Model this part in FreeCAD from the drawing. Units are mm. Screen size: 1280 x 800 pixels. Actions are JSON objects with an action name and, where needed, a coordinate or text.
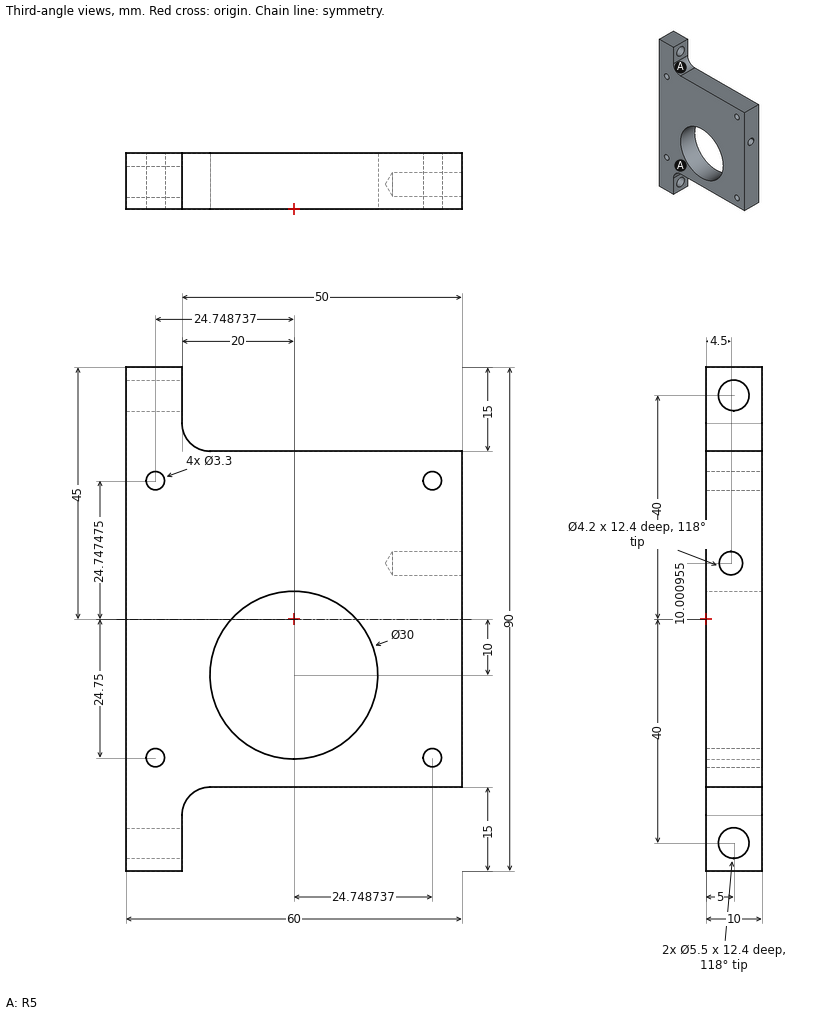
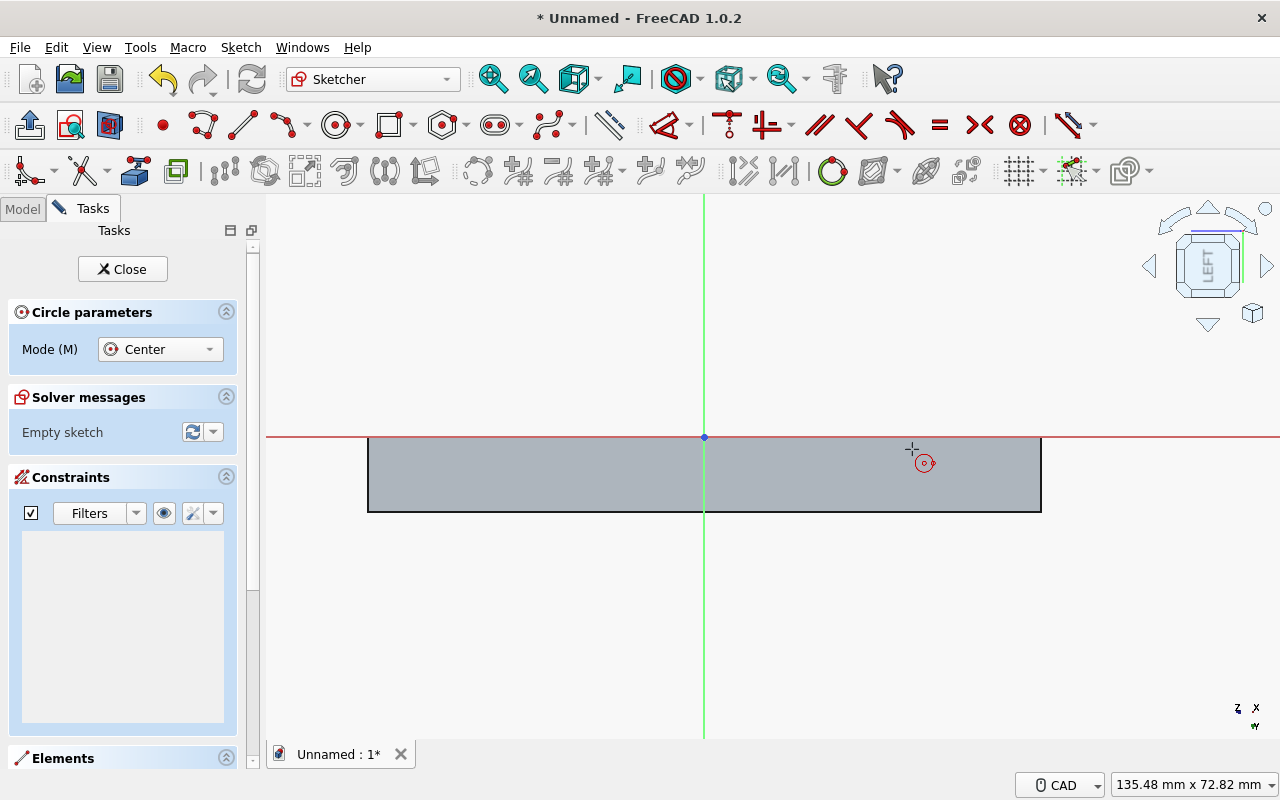
{"action": "left_click", "coordinate": [1004, 475]}
{"action": "mouse_move", "coordinate": [1018, 460]}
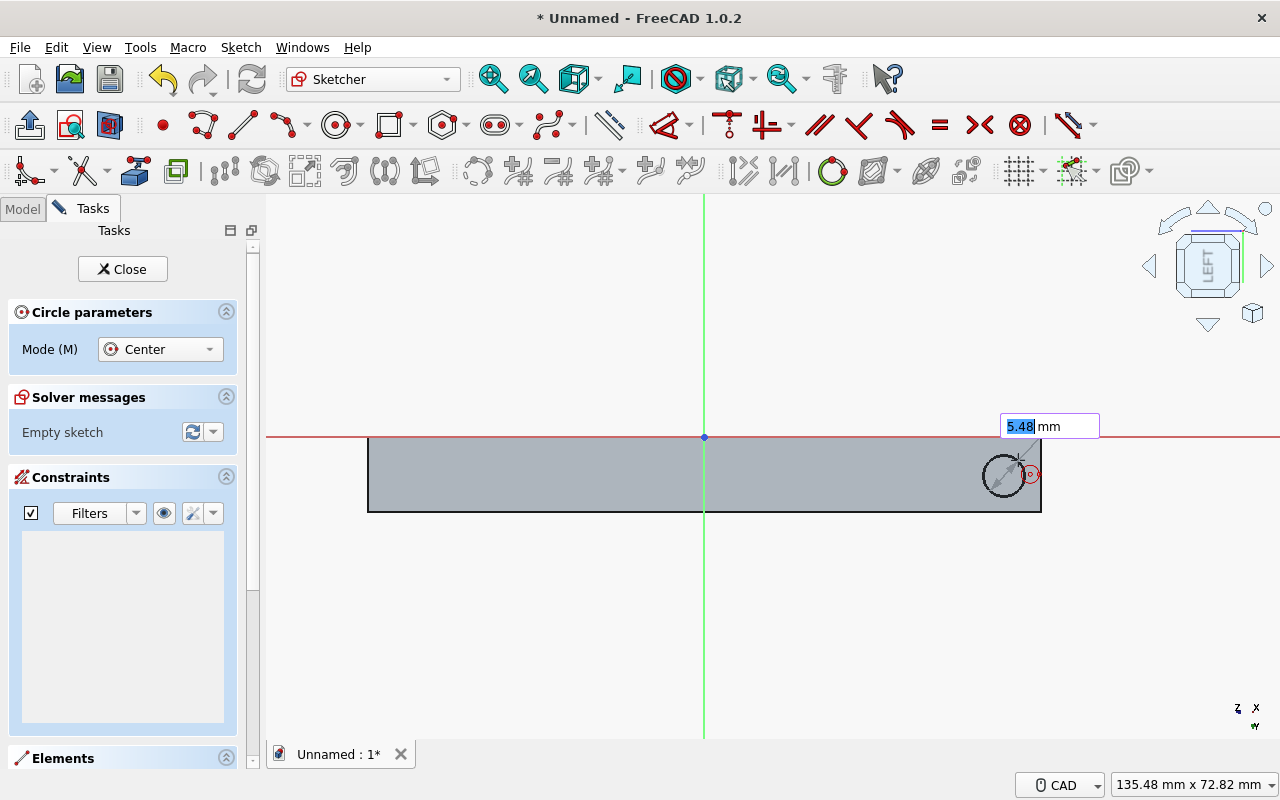
{"action": "type", "text": "5.5"}
{"action": "key", "text": "Return"}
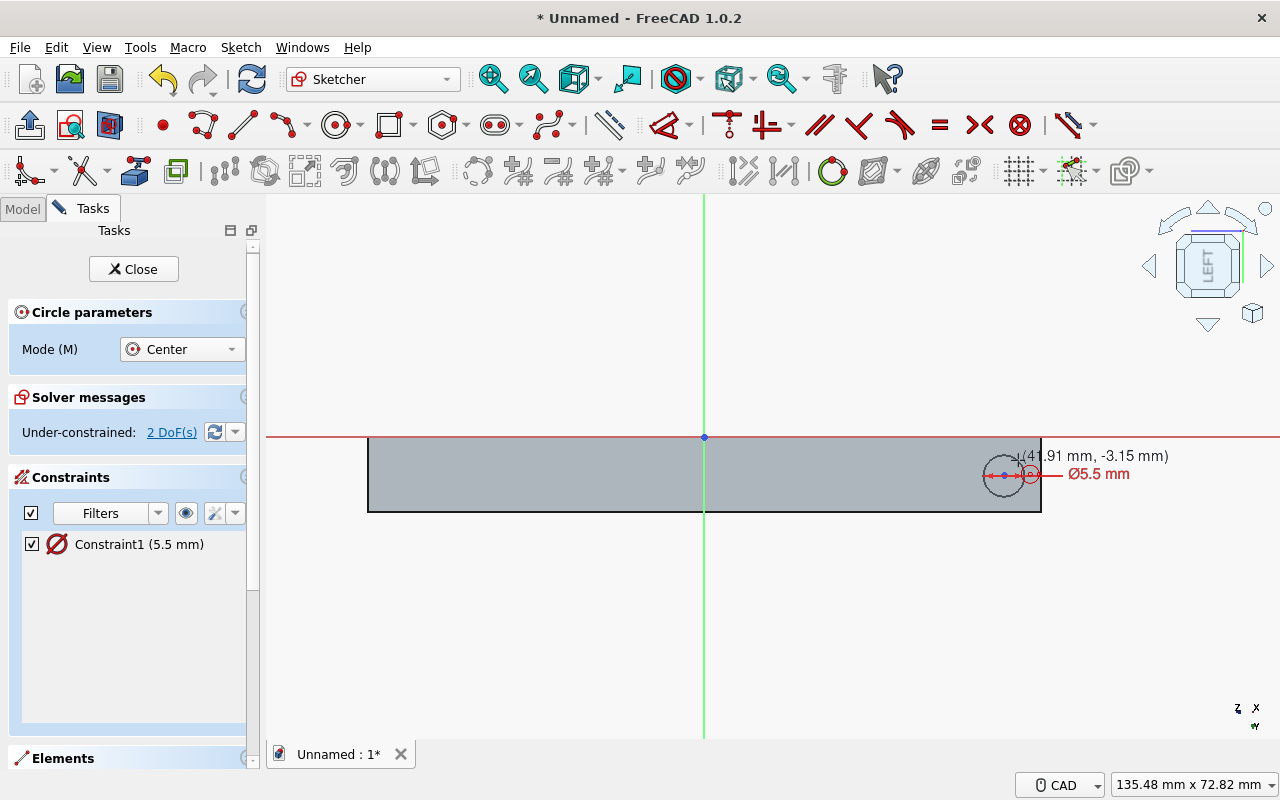
{"action": "left_click", "coordinate": [405, 475]}
{"action": "mouse_move", "coordinate": [419, 460]}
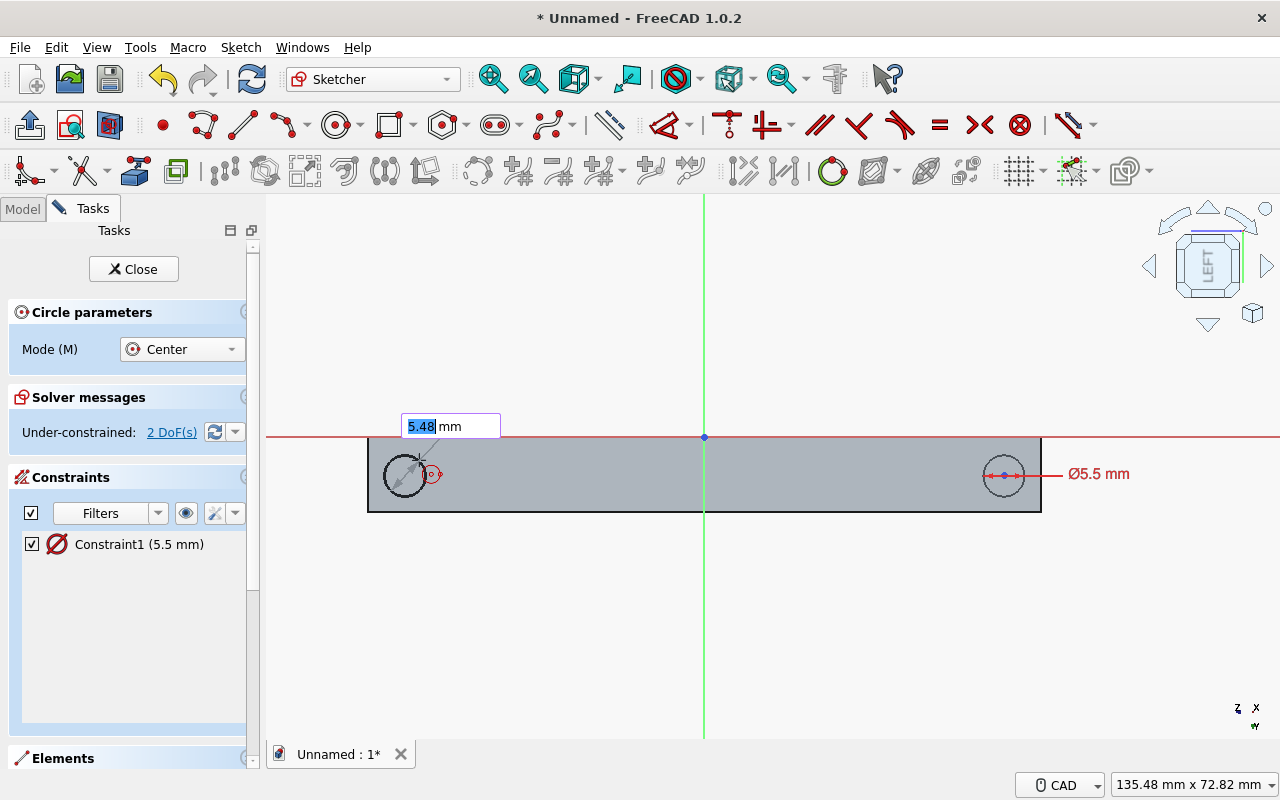
{"action": "type", "text": "5.5"}
{"action": "key", "text": "Return"}
{"action": "key", "text": "Escape"}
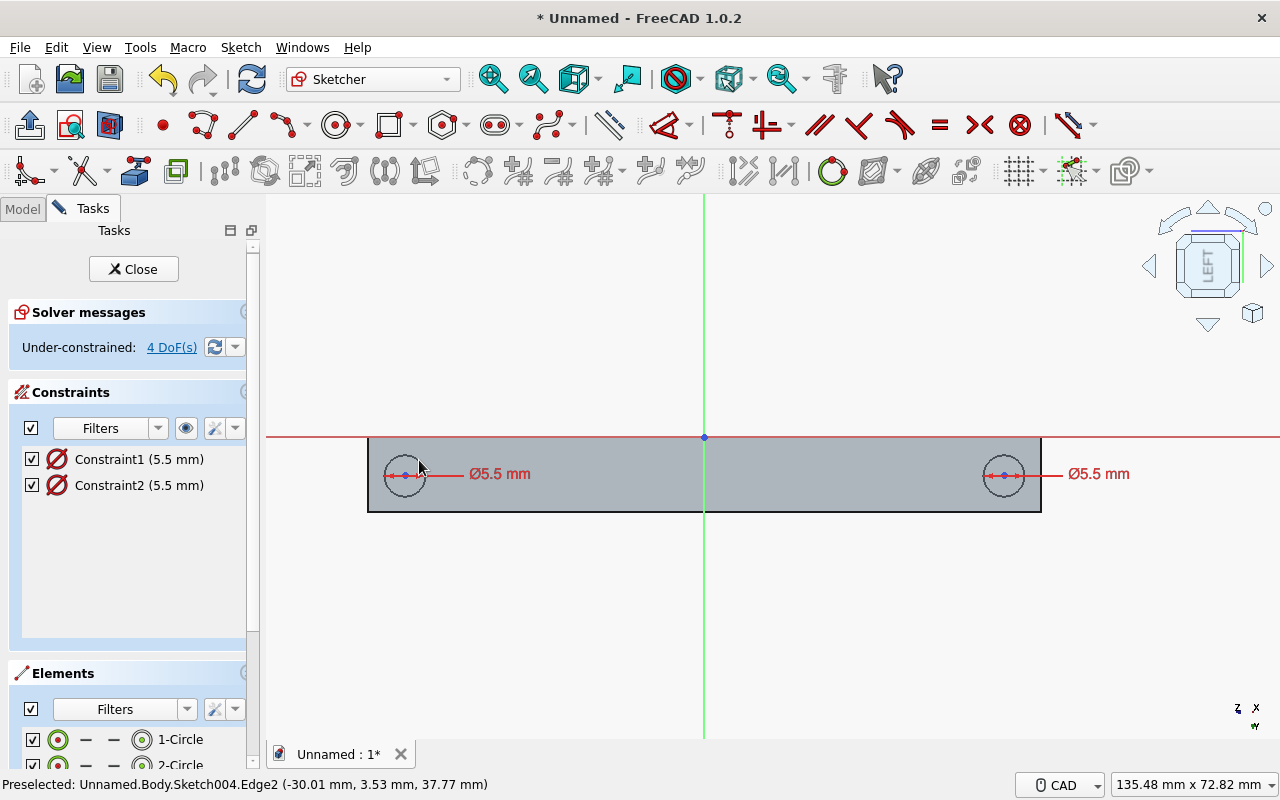
{"action": "left_click", "coordinate": [1004, 476]}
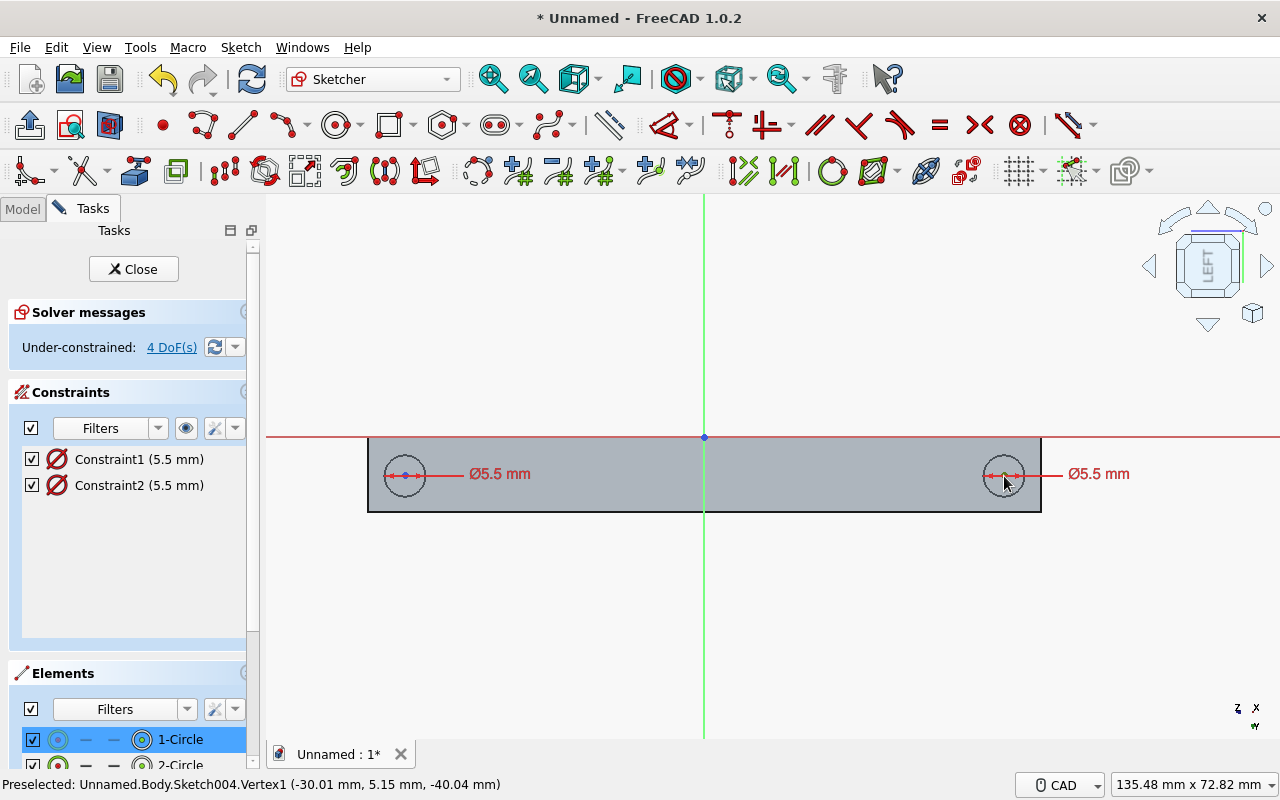
{"action": "left_click", "coordinate": [405, 476]}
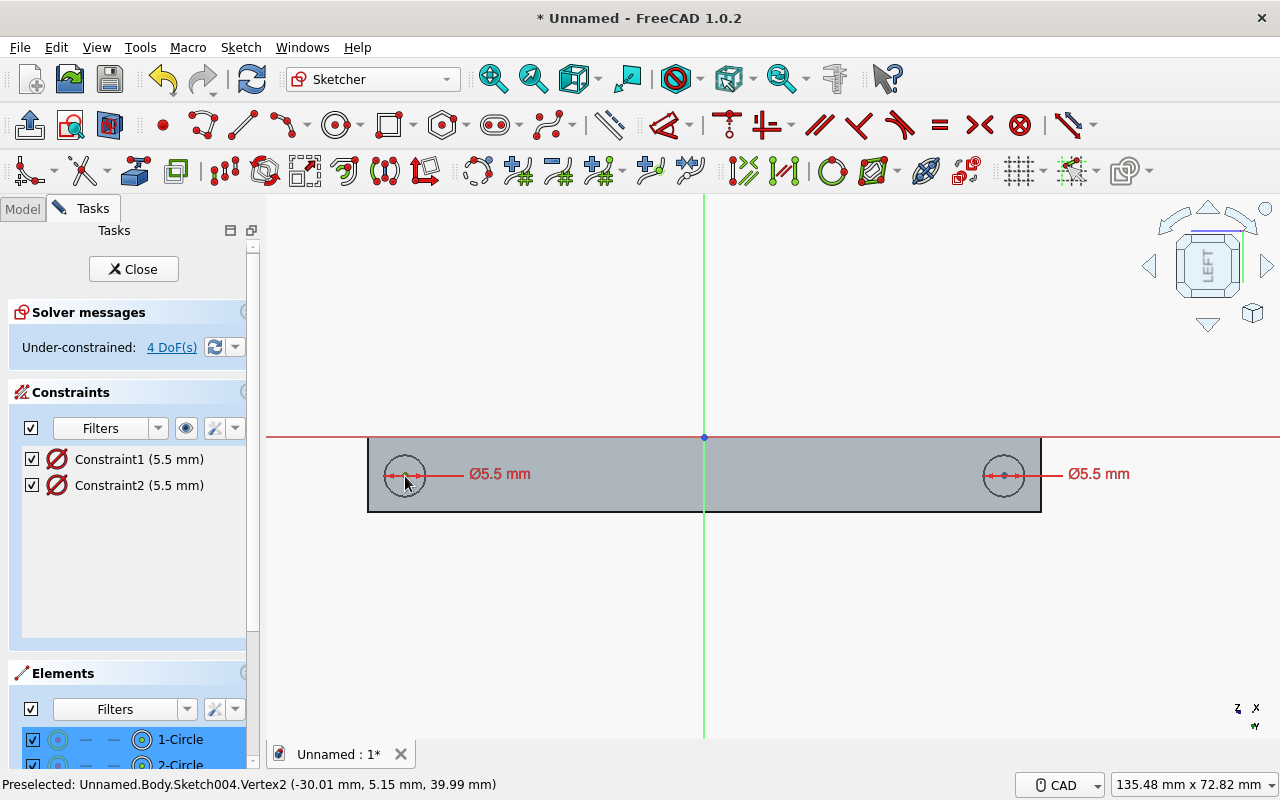
{"action": "key", "text": "h"}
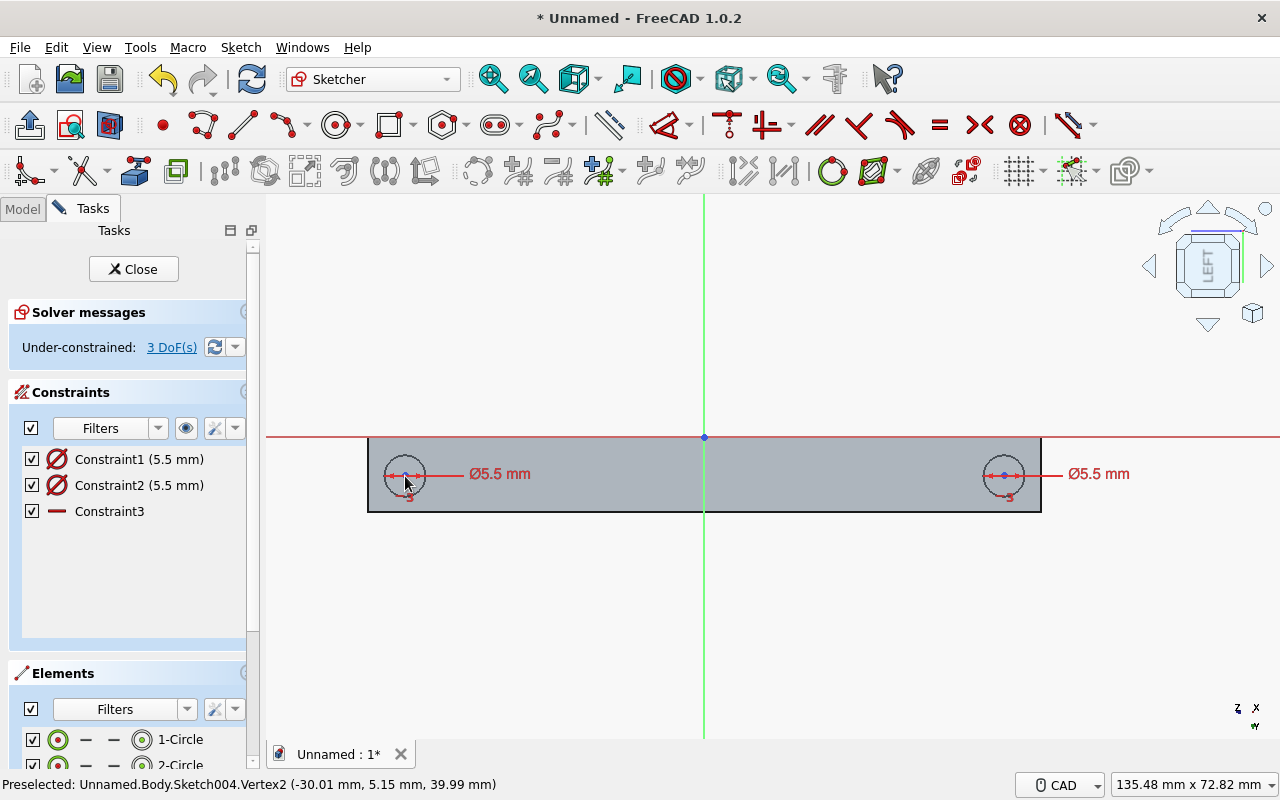
{"action": "left_click", "coordinate": [664, 126]}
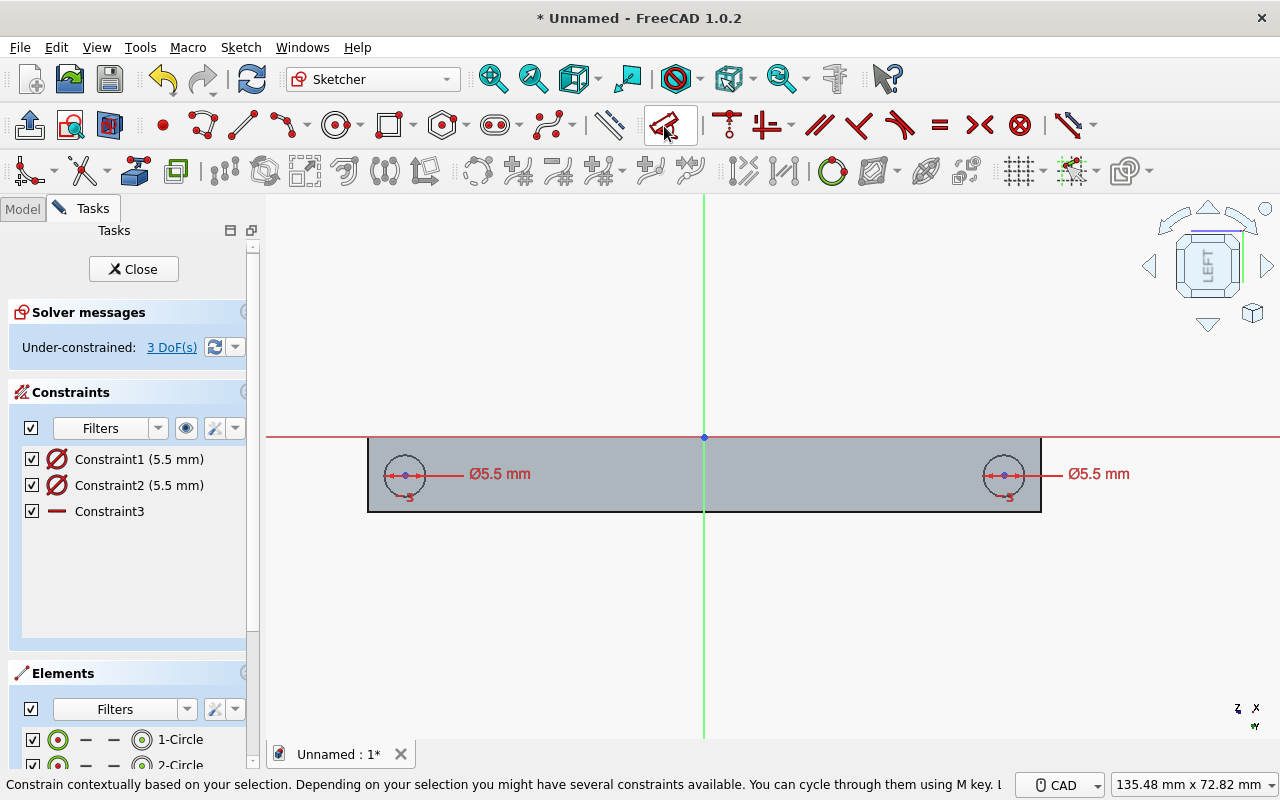
{"action": "left_click", "coordinate": [1004, 476]}
{"action": "left_click", "coordinate": [1038, 457]}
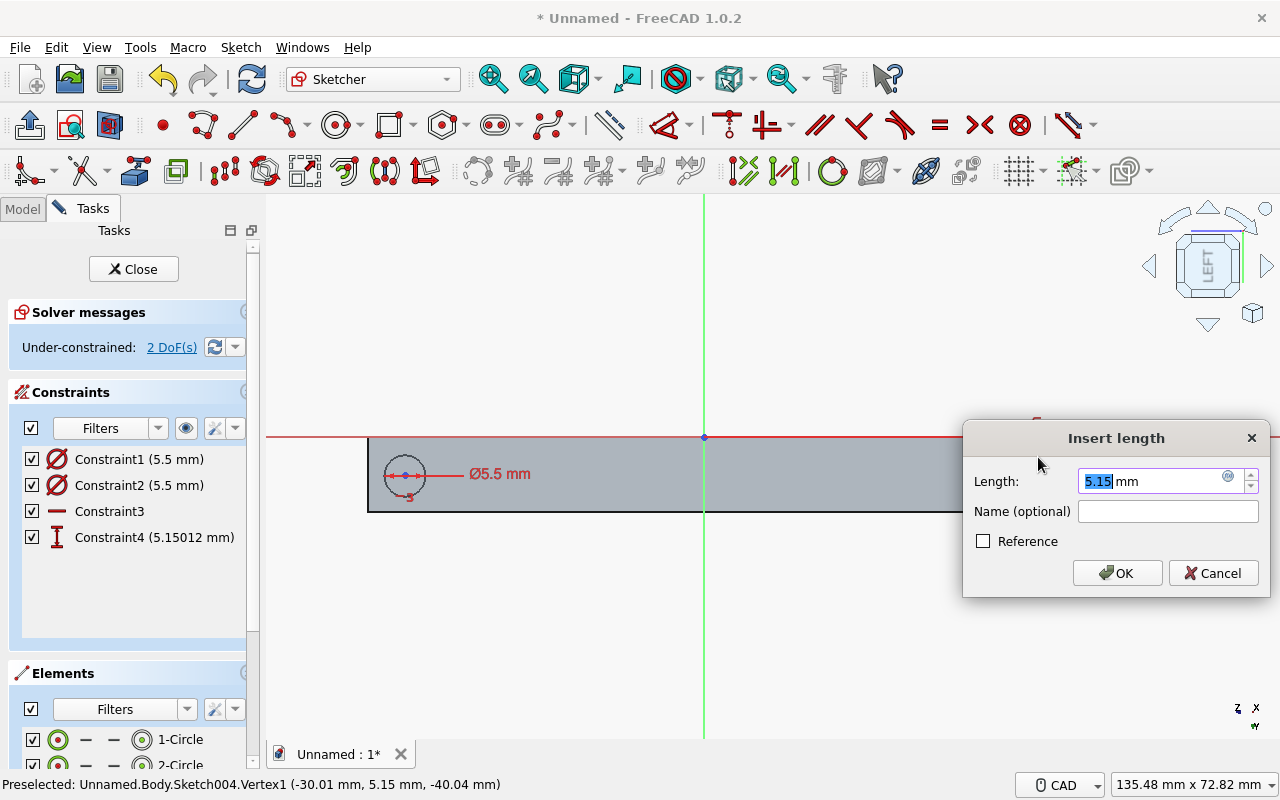
{"action": "type", "text": "5"}
{"action": "key", "text": "Return"}